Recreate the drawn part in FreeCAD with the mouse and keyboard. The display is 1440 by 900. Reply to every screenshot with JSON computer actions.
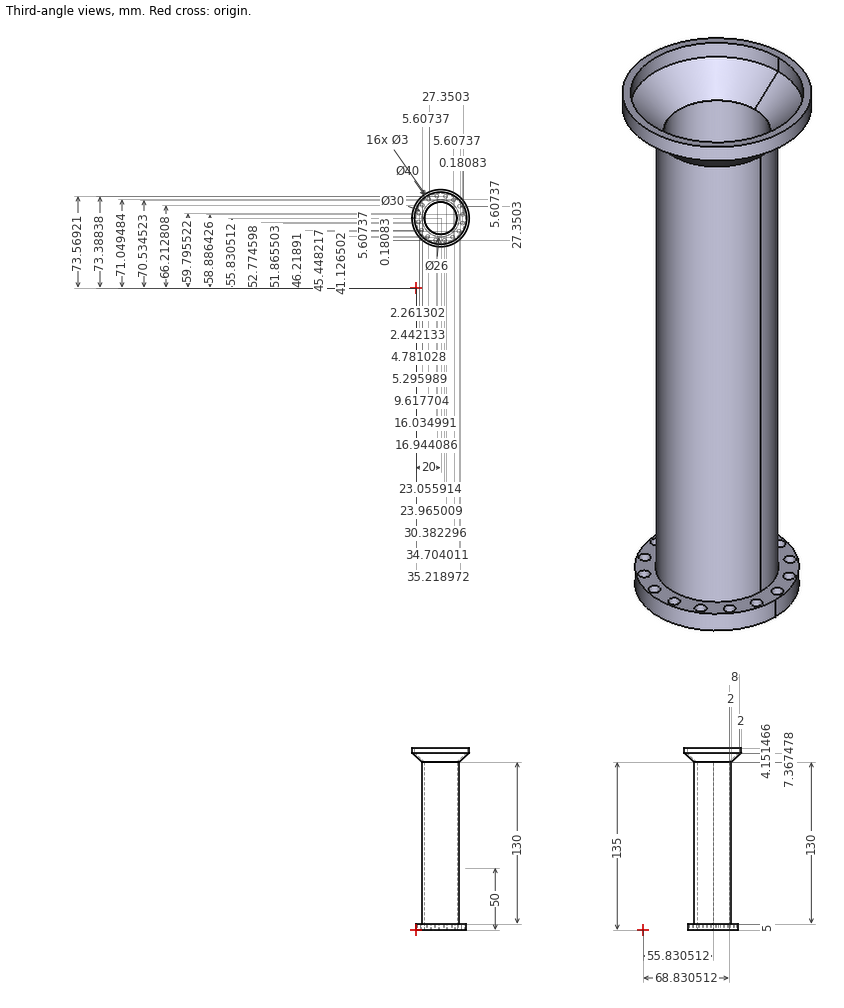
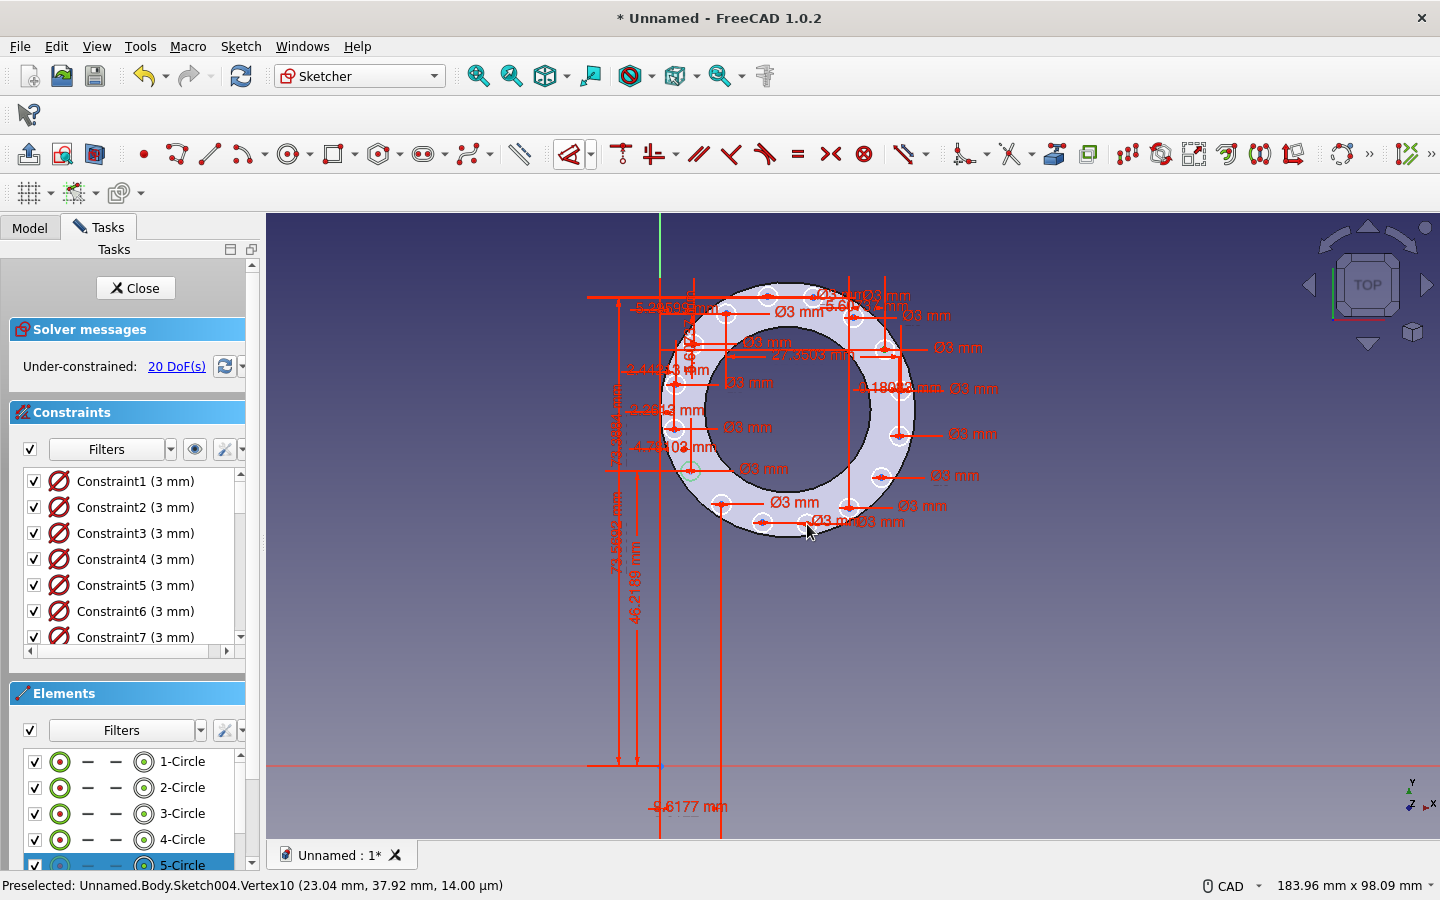
{"action": "left_click", "coordinate": [590, 154]}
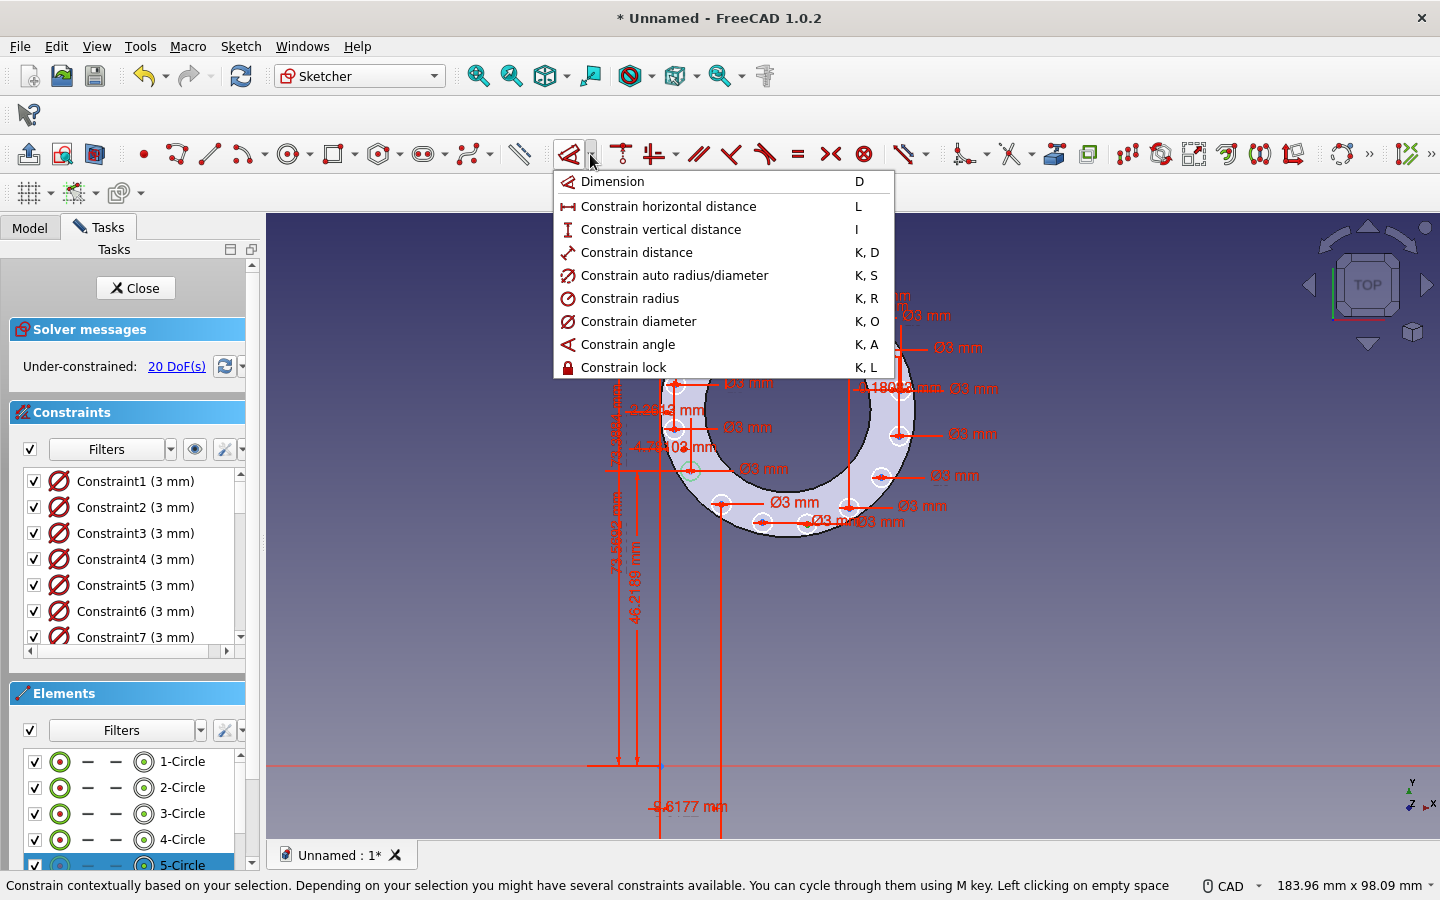
{"action": "left_click", "coordinate": [724, 230]}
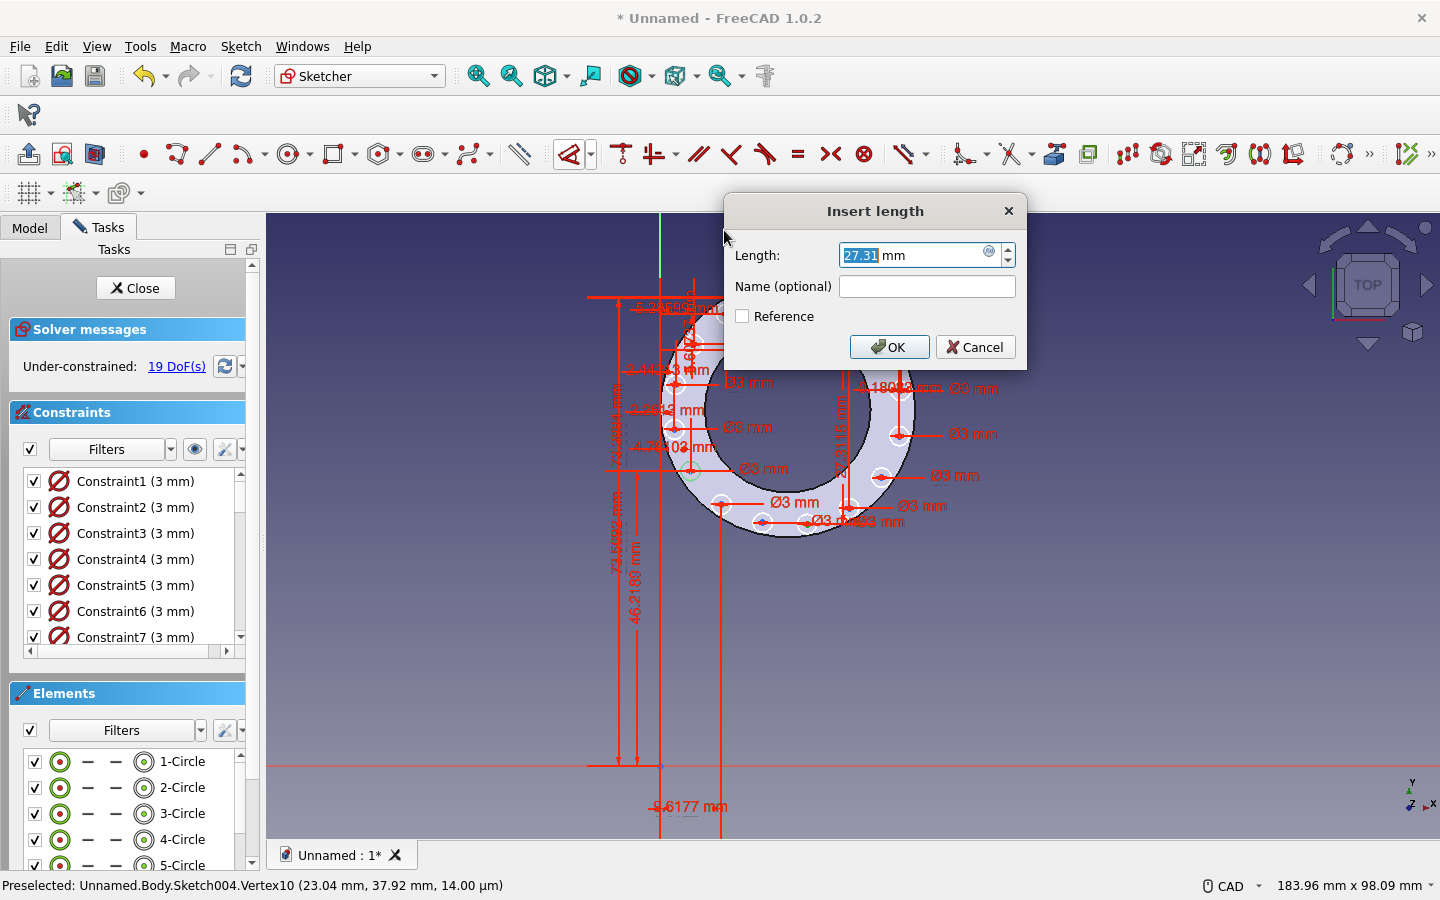
{"action": "type", "text": "27.3503"}
{"action": "key", "text": "Return"}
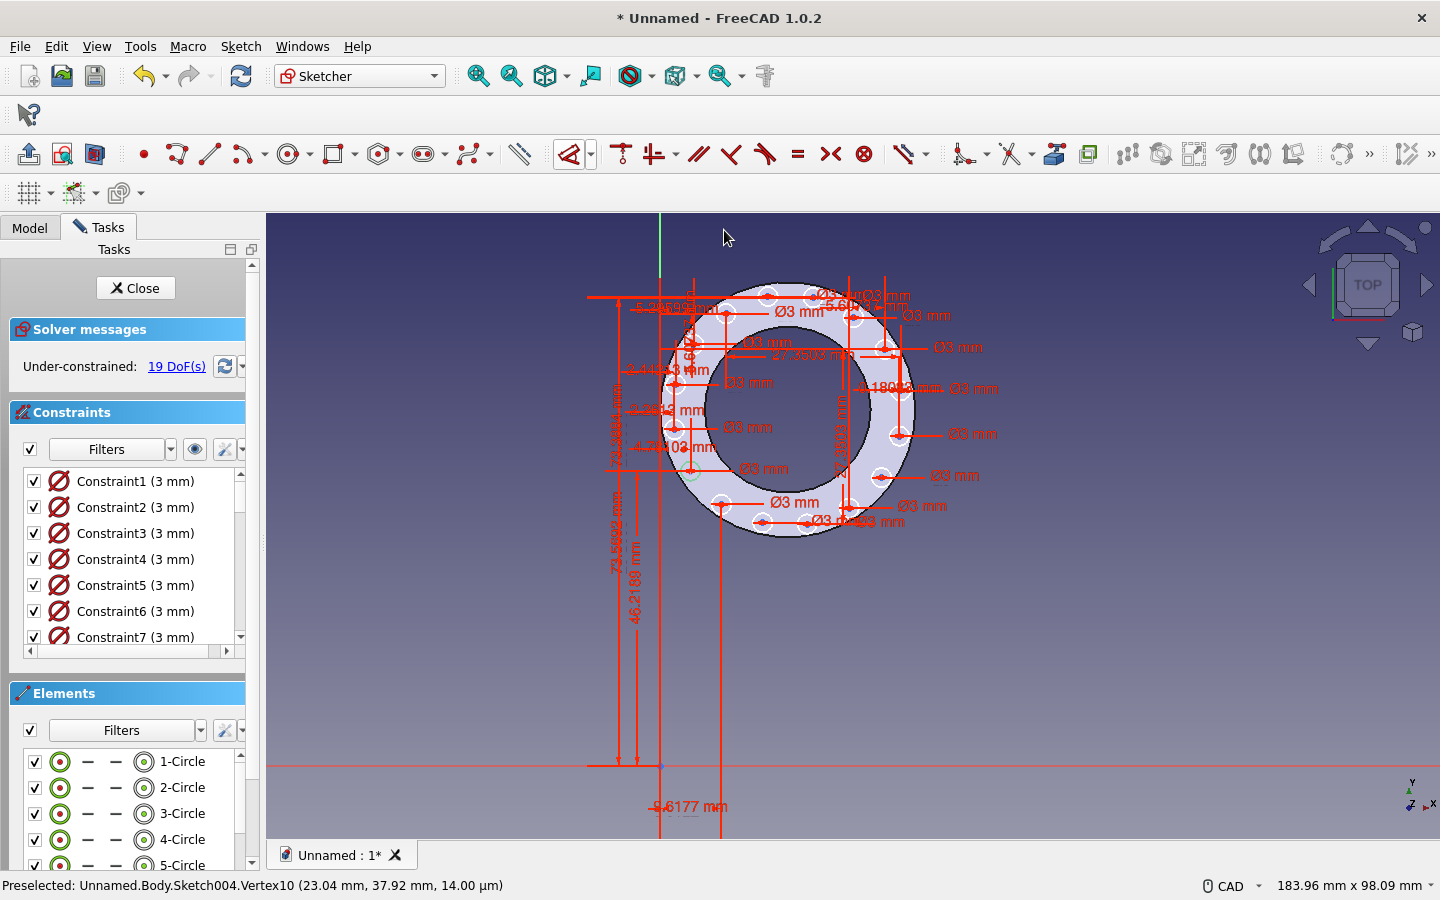
{"action": "scroll", "coordinate": [807, 524], "scroll_direction": "up", "scroll_amount": 18}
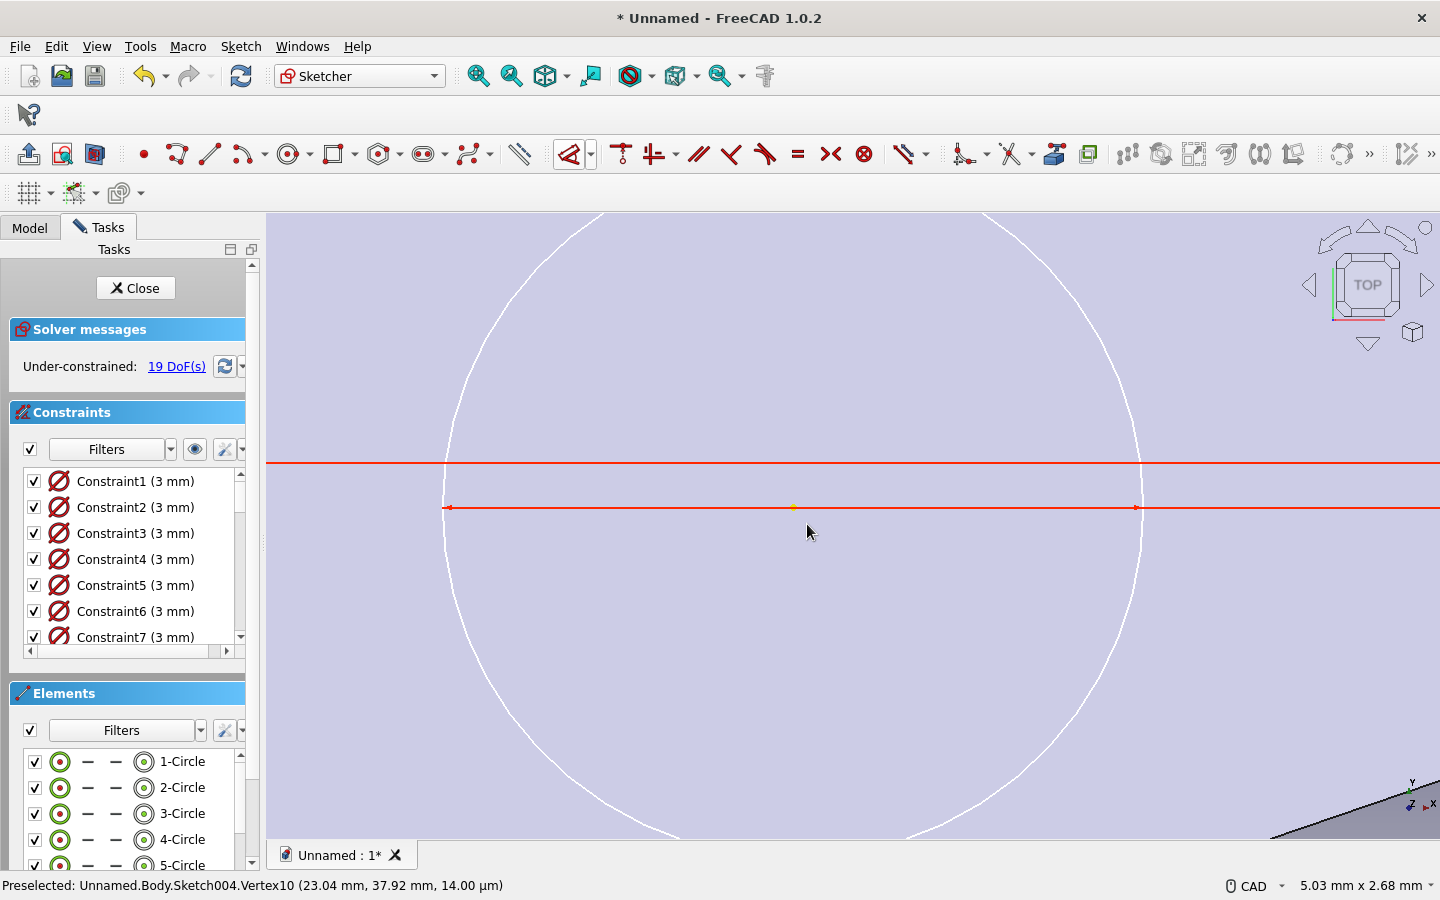
{"action": "left_click", "coordinate": [793, 508]}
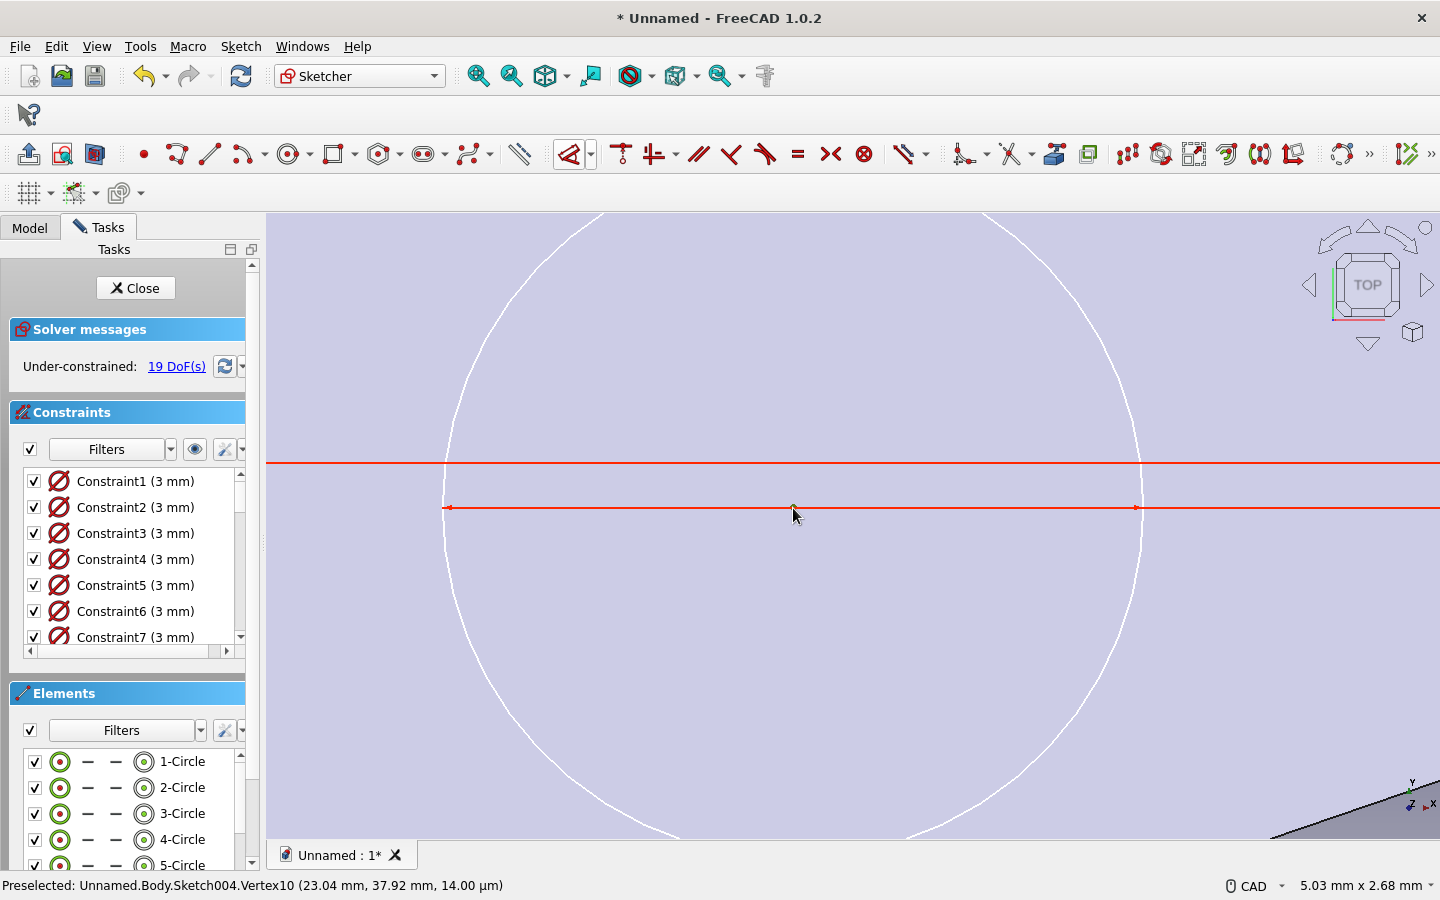
{"action": "scroll", "coordinate": [807, 524], "scroll_direction": "down", "scroll_amount": 18}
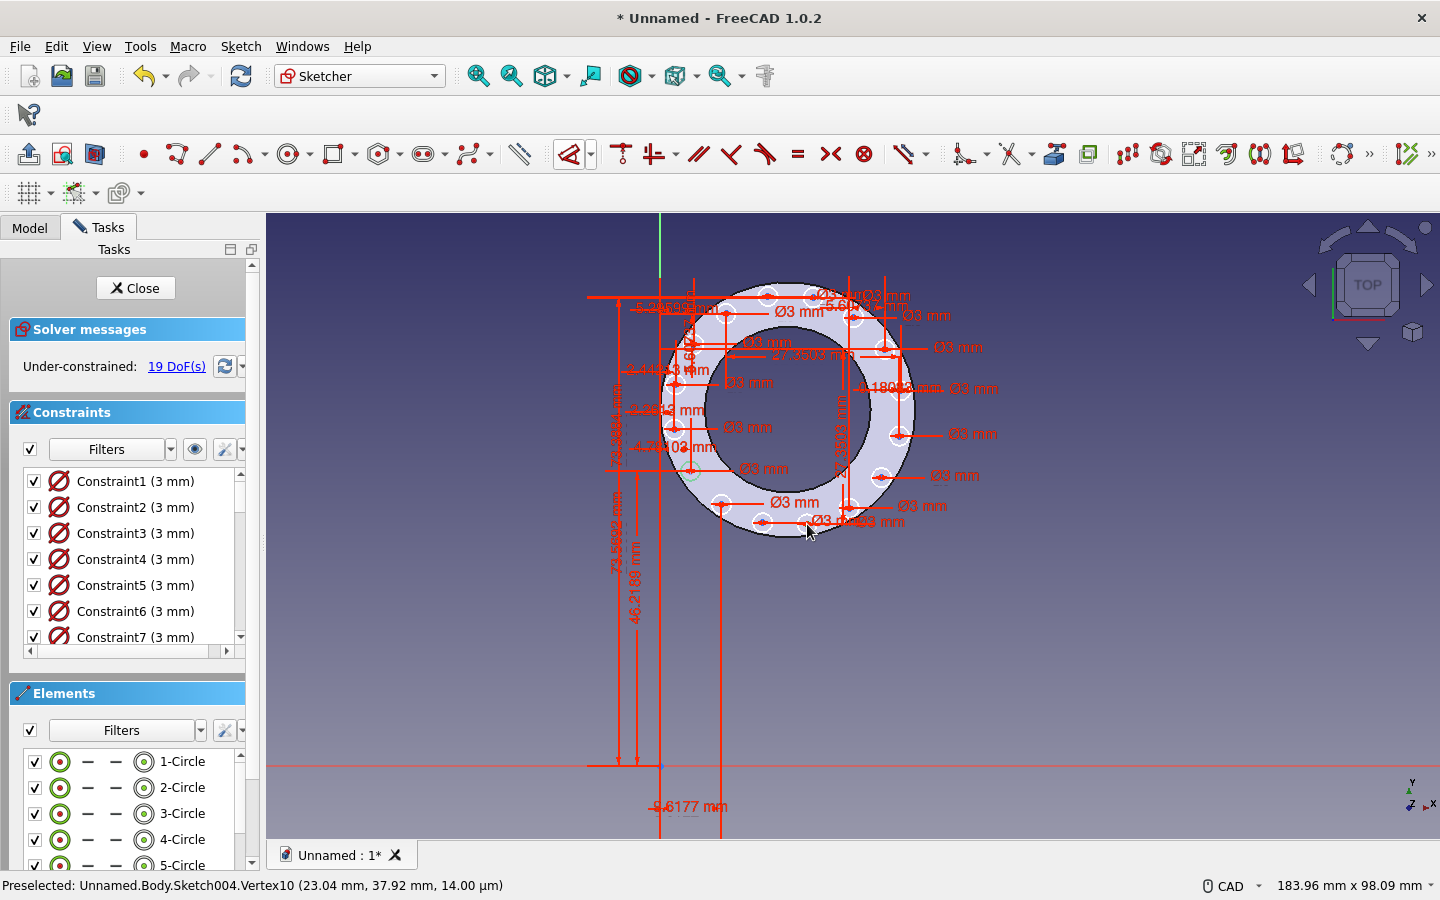
{"action": "scroll", "coordinate": [763, 523], "scroll_direction": "up", "scroll_amount": 18}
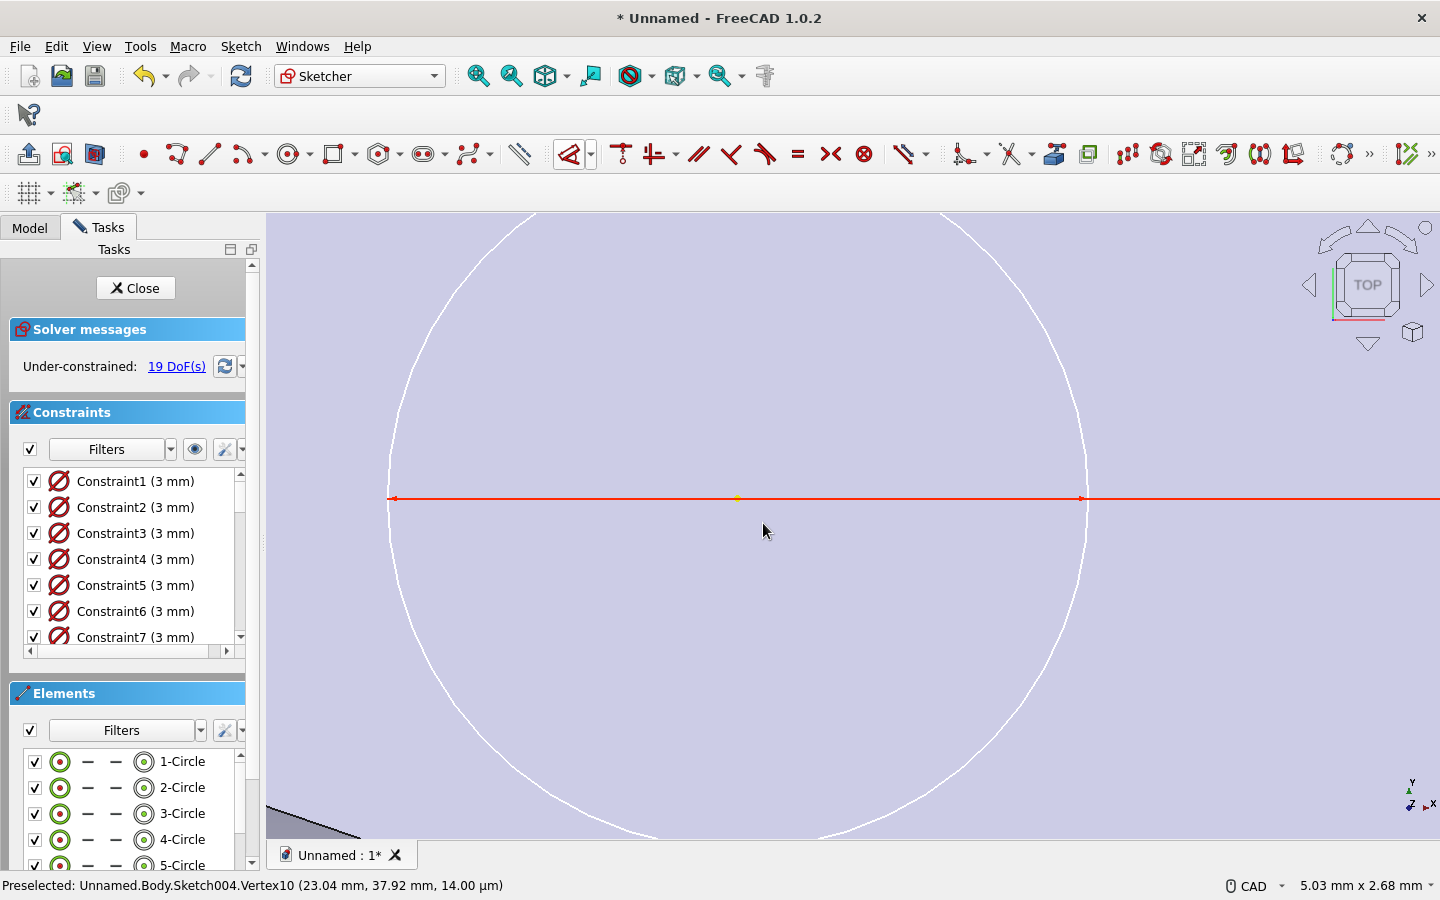
{"action": "left_click", "coordinate": [738, 499]}